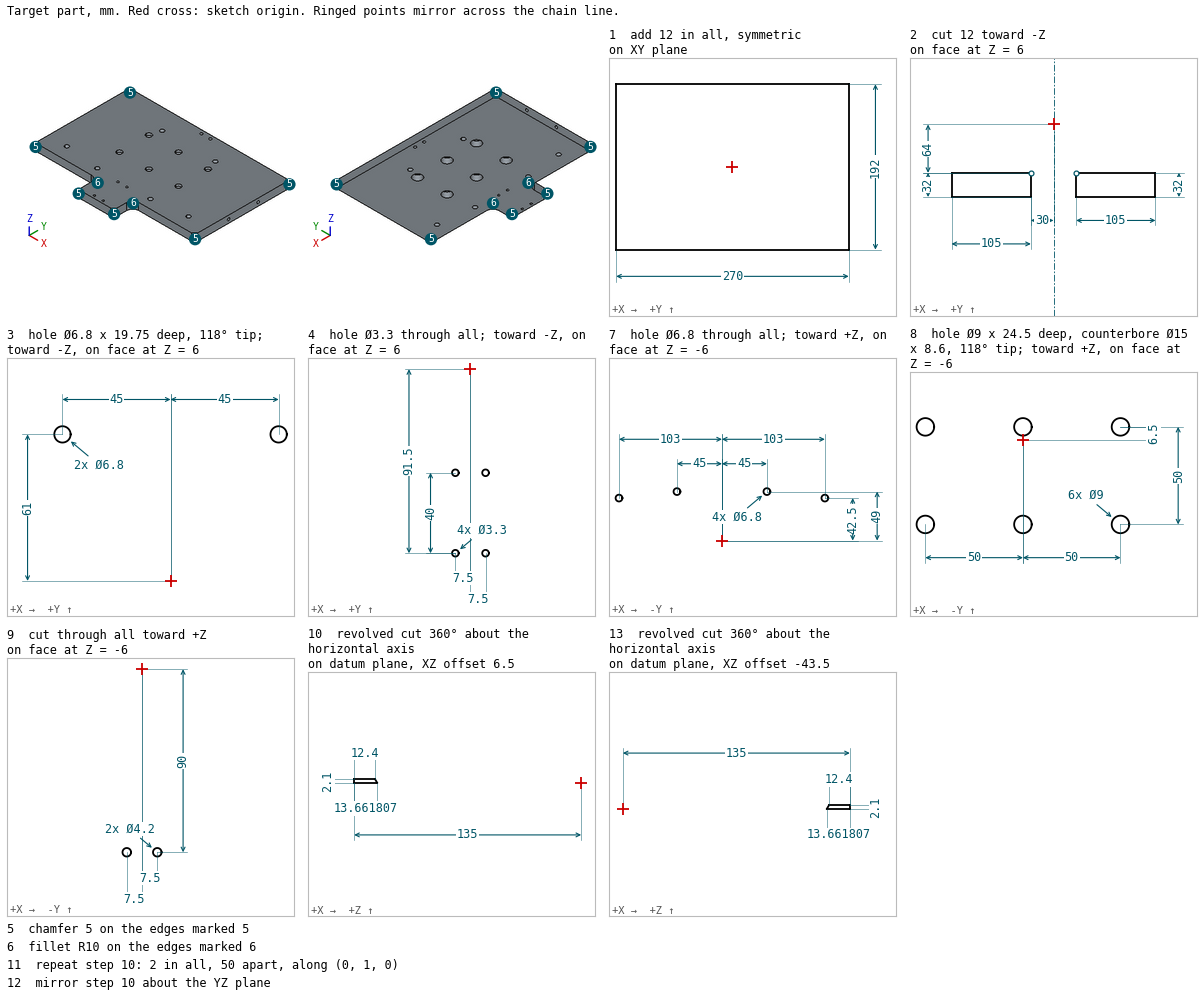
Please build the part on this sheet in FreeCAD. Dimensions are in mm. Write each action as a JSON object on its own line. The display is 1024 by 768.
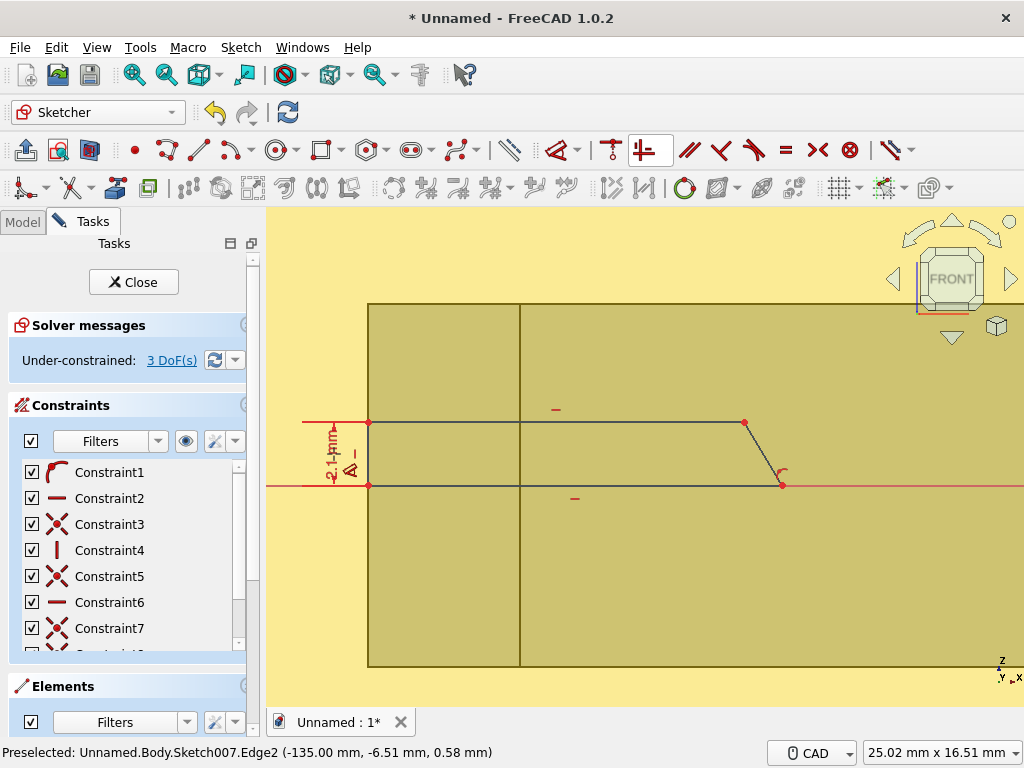
{"action": "left_click", "coordinate": [481, 422]}
{"action": "left_click", "coordinate": [556, 388]}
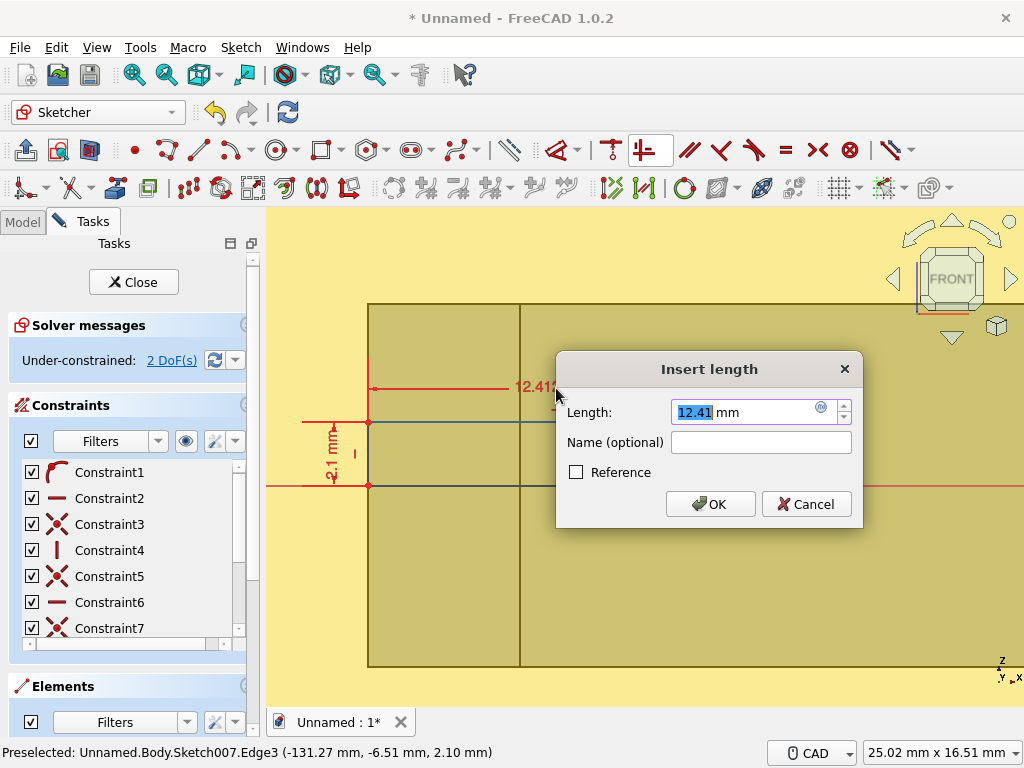
{"action": "type", "text": "12.4"}
{"action": "key", "text": "Return"}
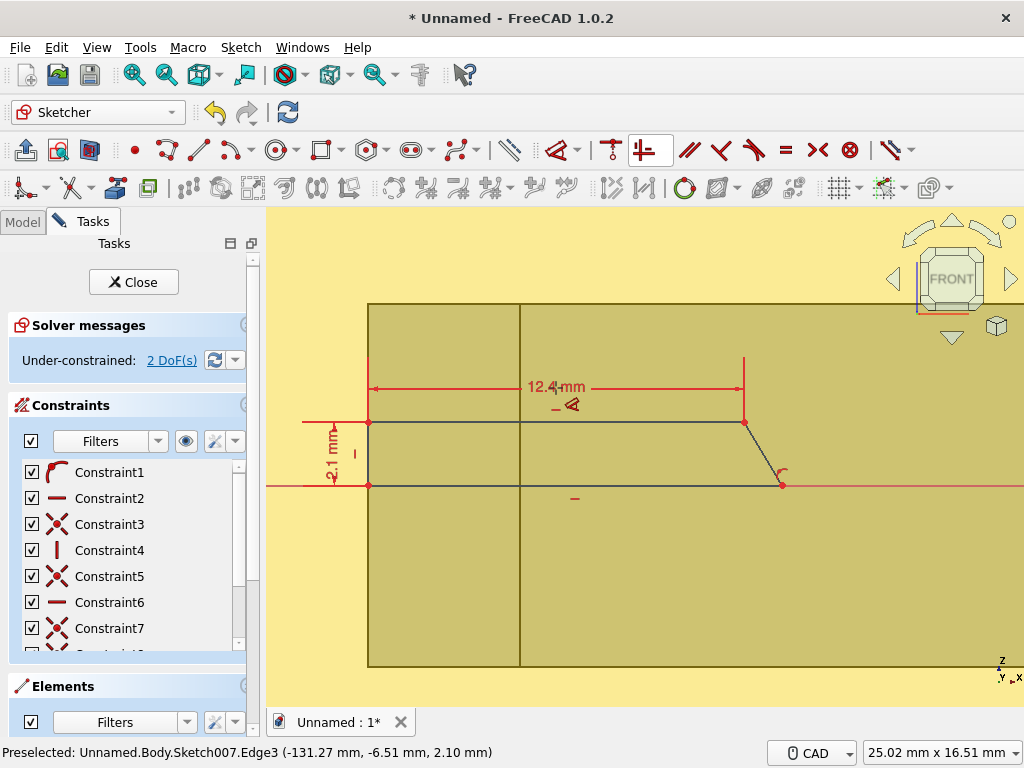
{"action": "left_click", "coordinate": [368, 486]}
{"action": "left_click", "coordinate": [614, 520]}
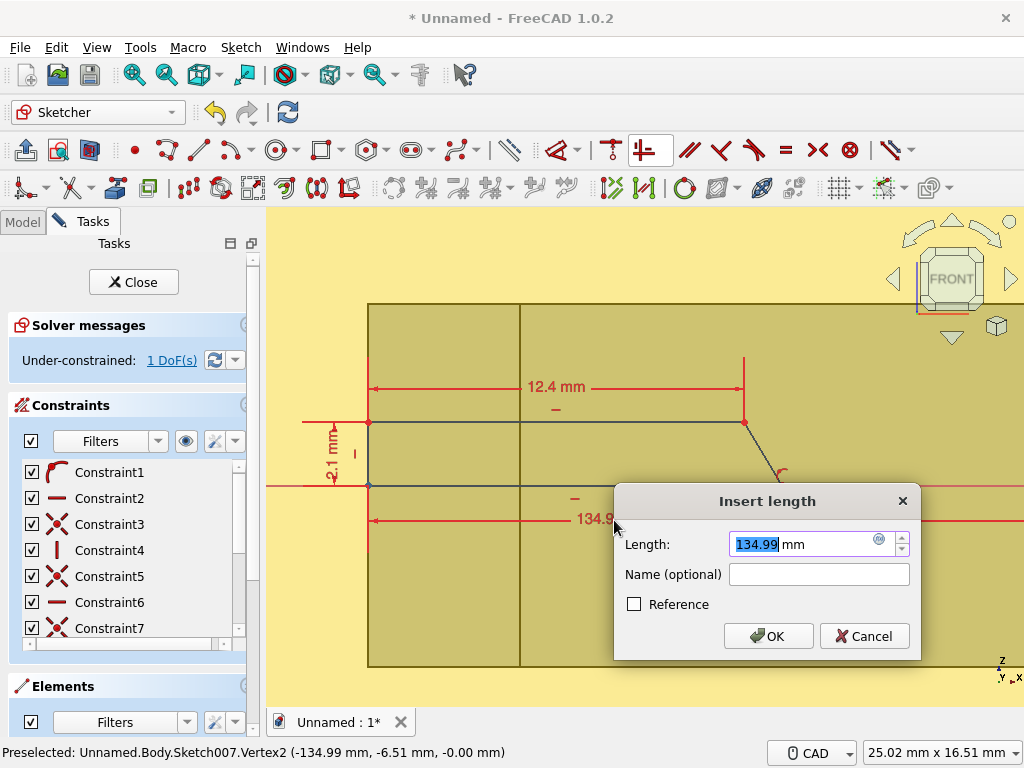
{"action": "type", "text": "135"}
{"action": "key", "text": "Return"}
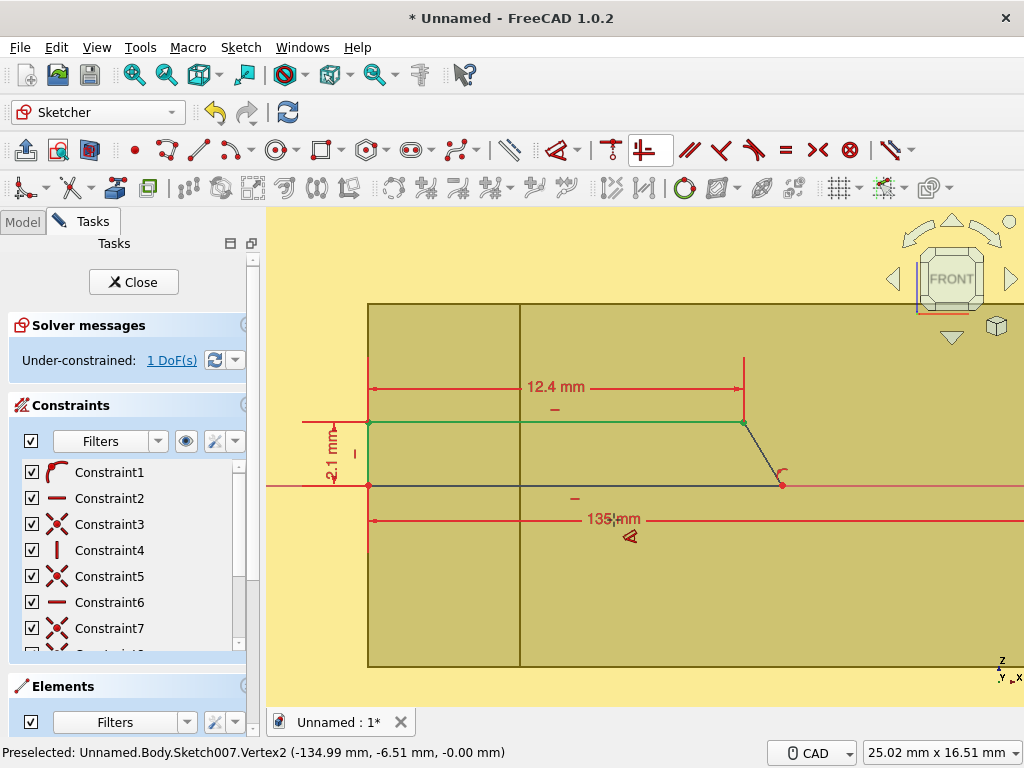
{"action": "left_click", "coordinate": [658, 486]}
{"action": "left_click", "coordinate": [480, 520]}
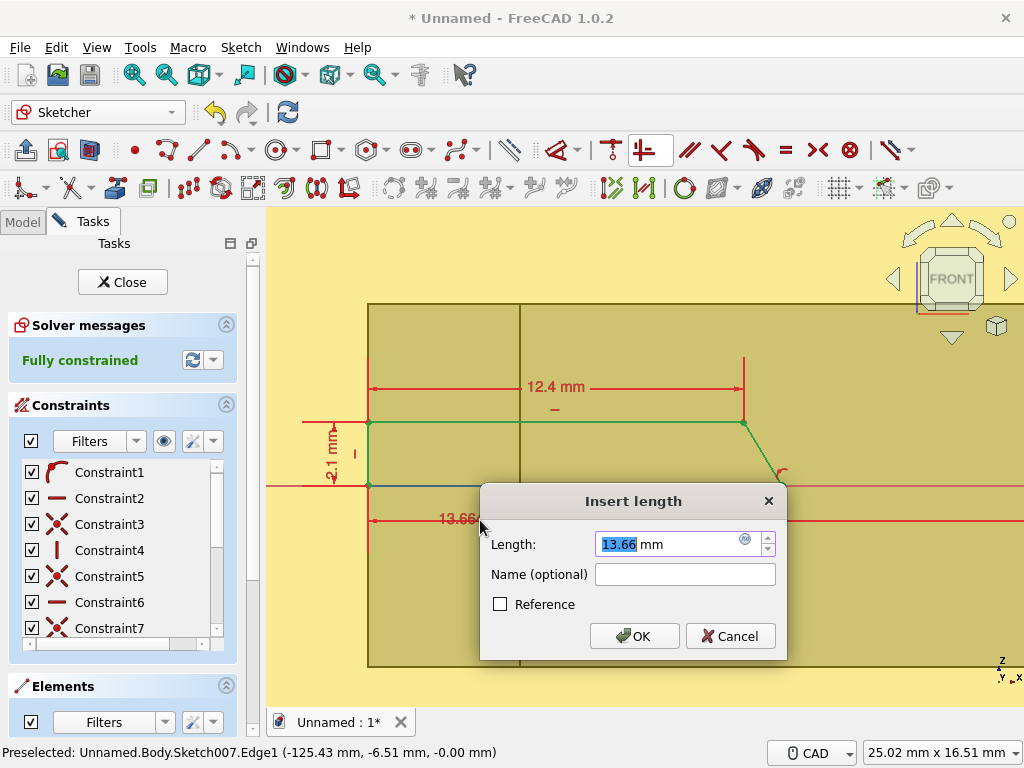
{"action": "type", "text": "13.661807"}
{"action": "key", "text": "Return"}
{"action": "key", "text": "Escape"}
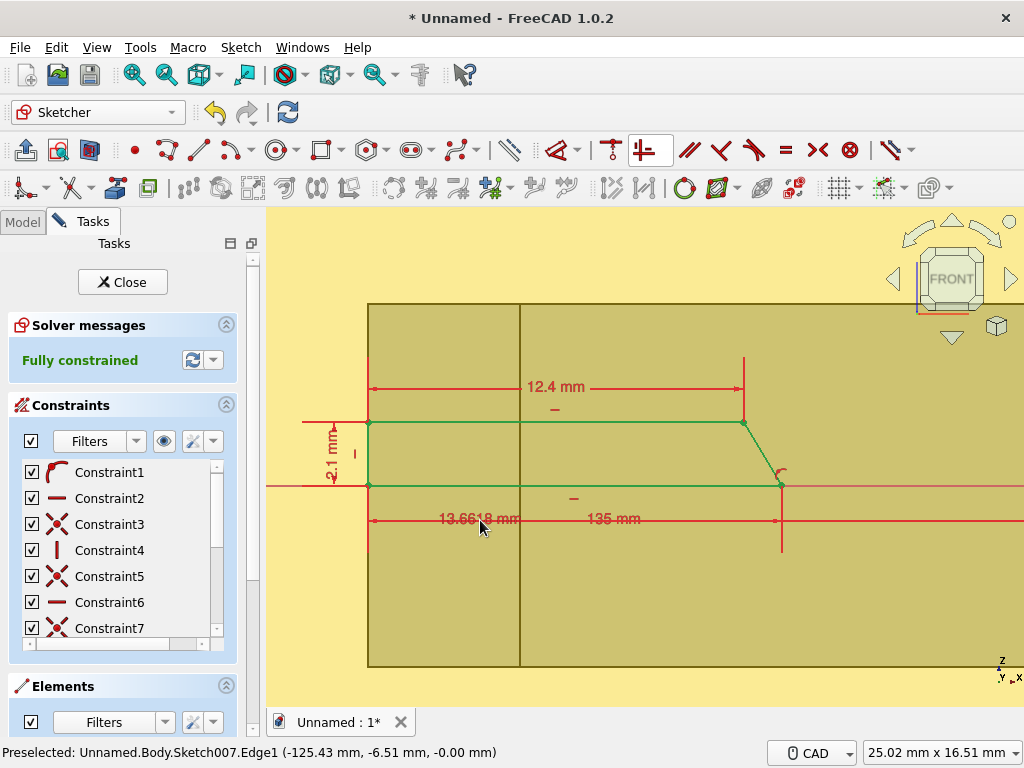
{"action": "left_click", "coordinate": [123, 282]}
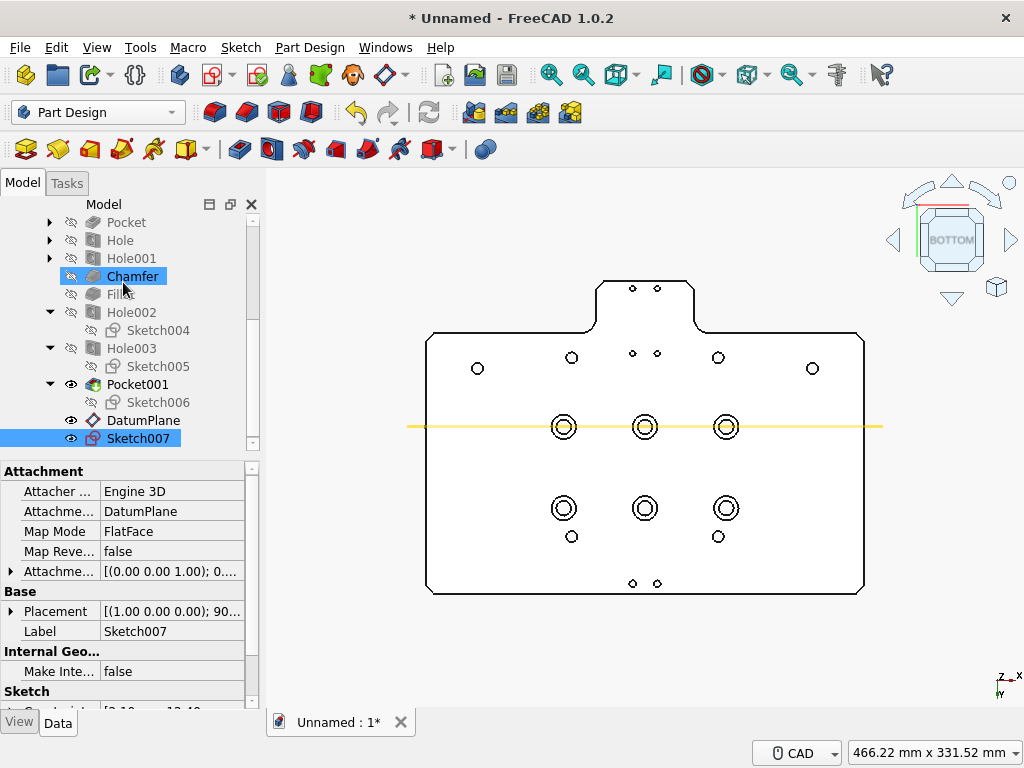
{"action": "left_click", "coordinate": [304, 150]}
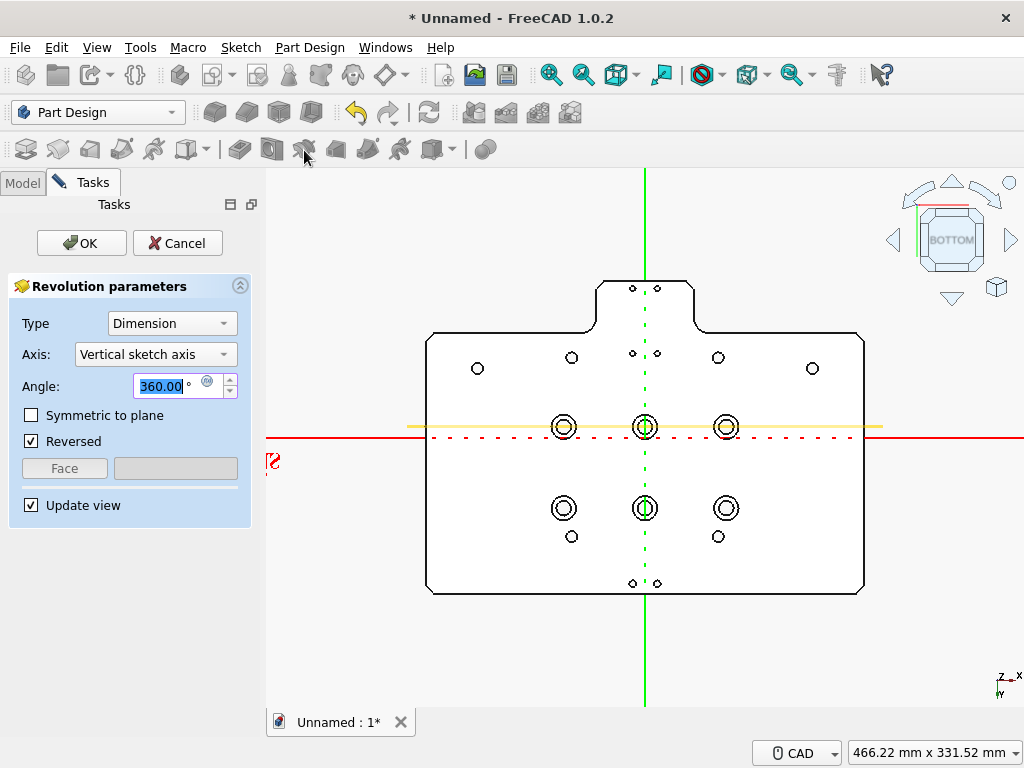
{"action": "left_click", "coordinate": [156, 354]}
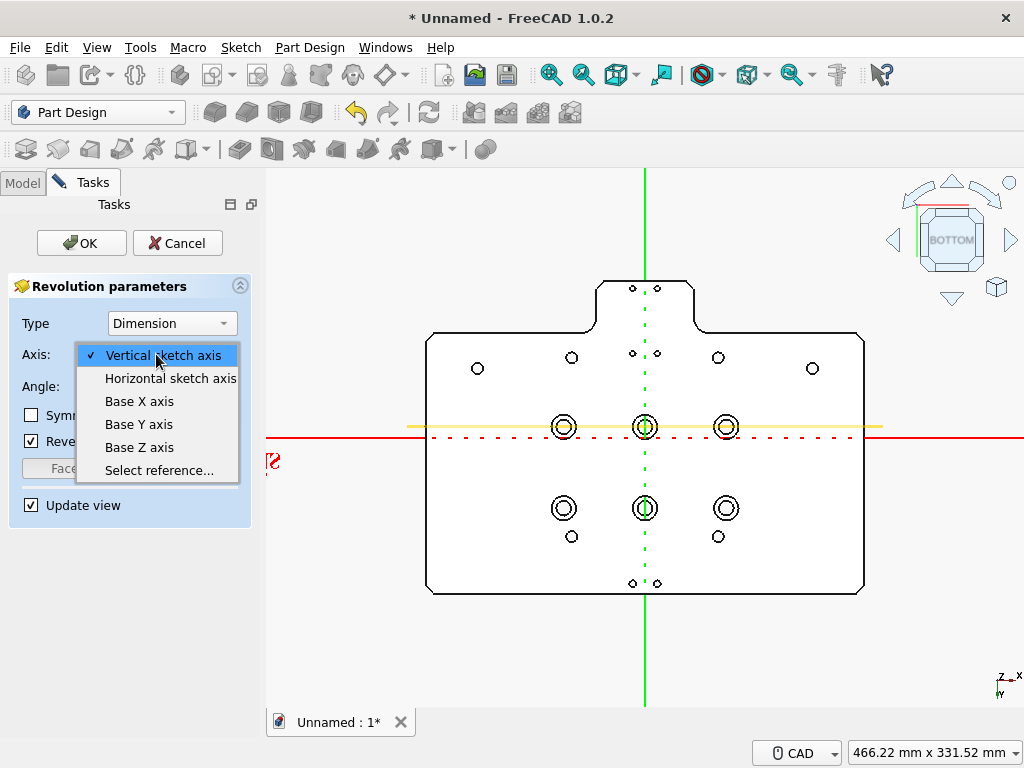
{"action": "left_click", "coordinate": [156, 378]}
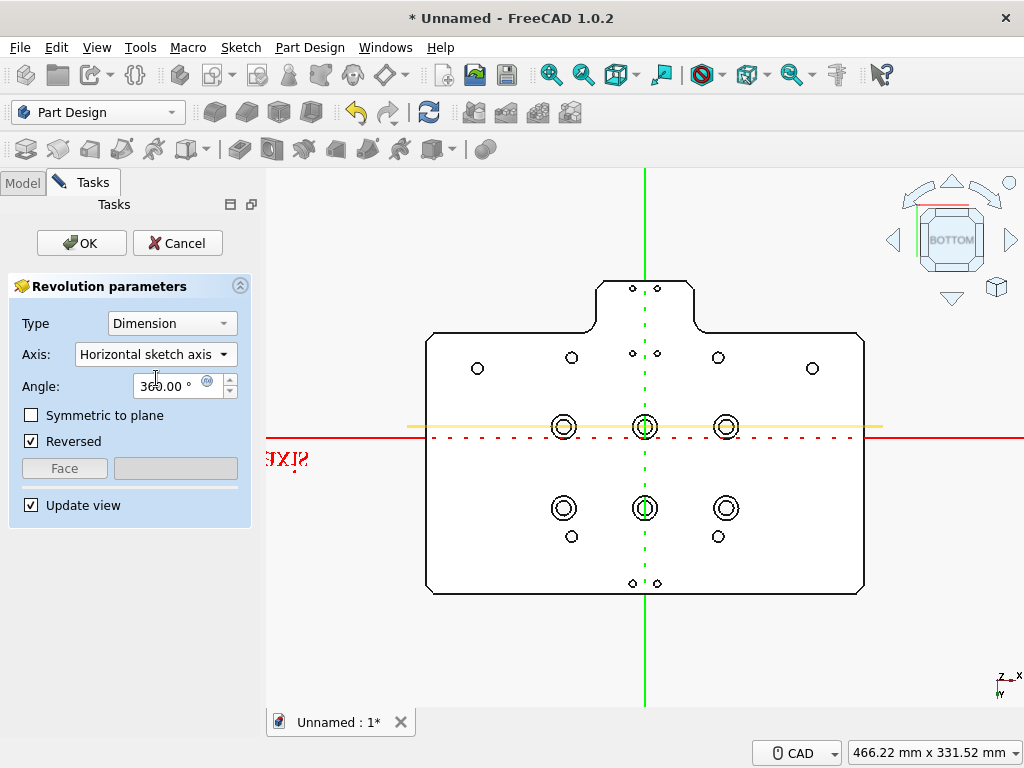
{"action": "left_click", "coordinate": [82, 243]}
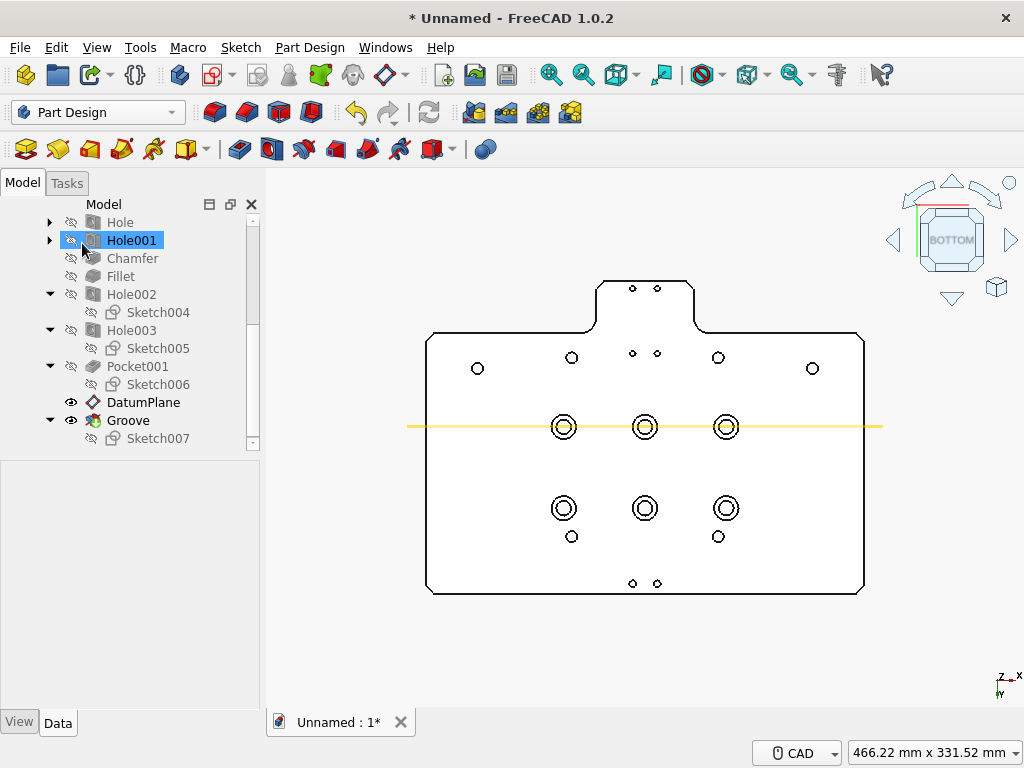
{"action": "left_click", "coordinate": [116, 402]}
{"action": "key", "text": "space"}